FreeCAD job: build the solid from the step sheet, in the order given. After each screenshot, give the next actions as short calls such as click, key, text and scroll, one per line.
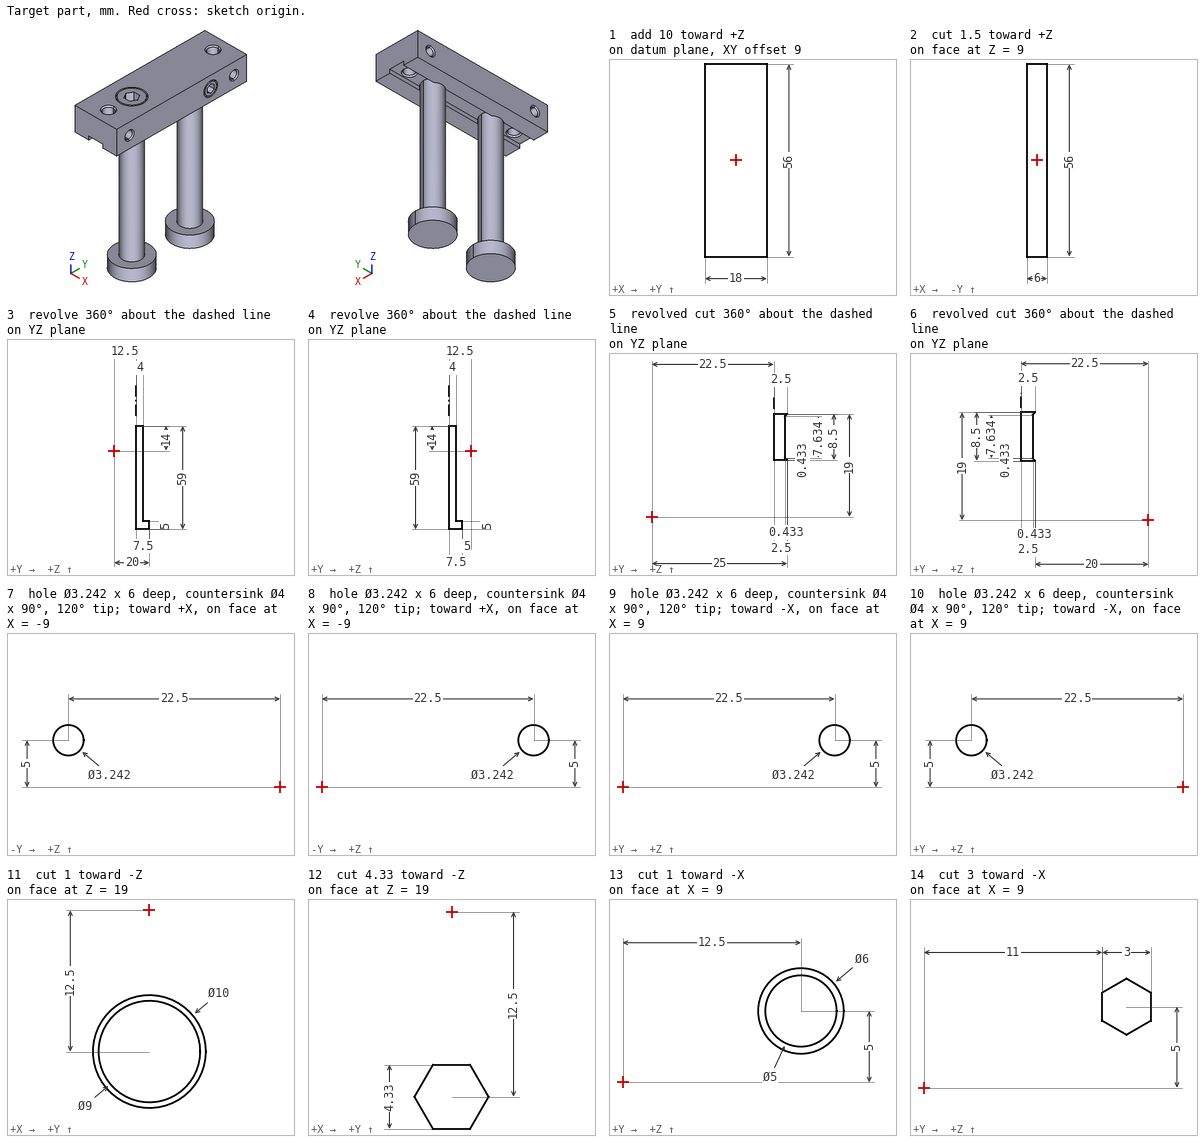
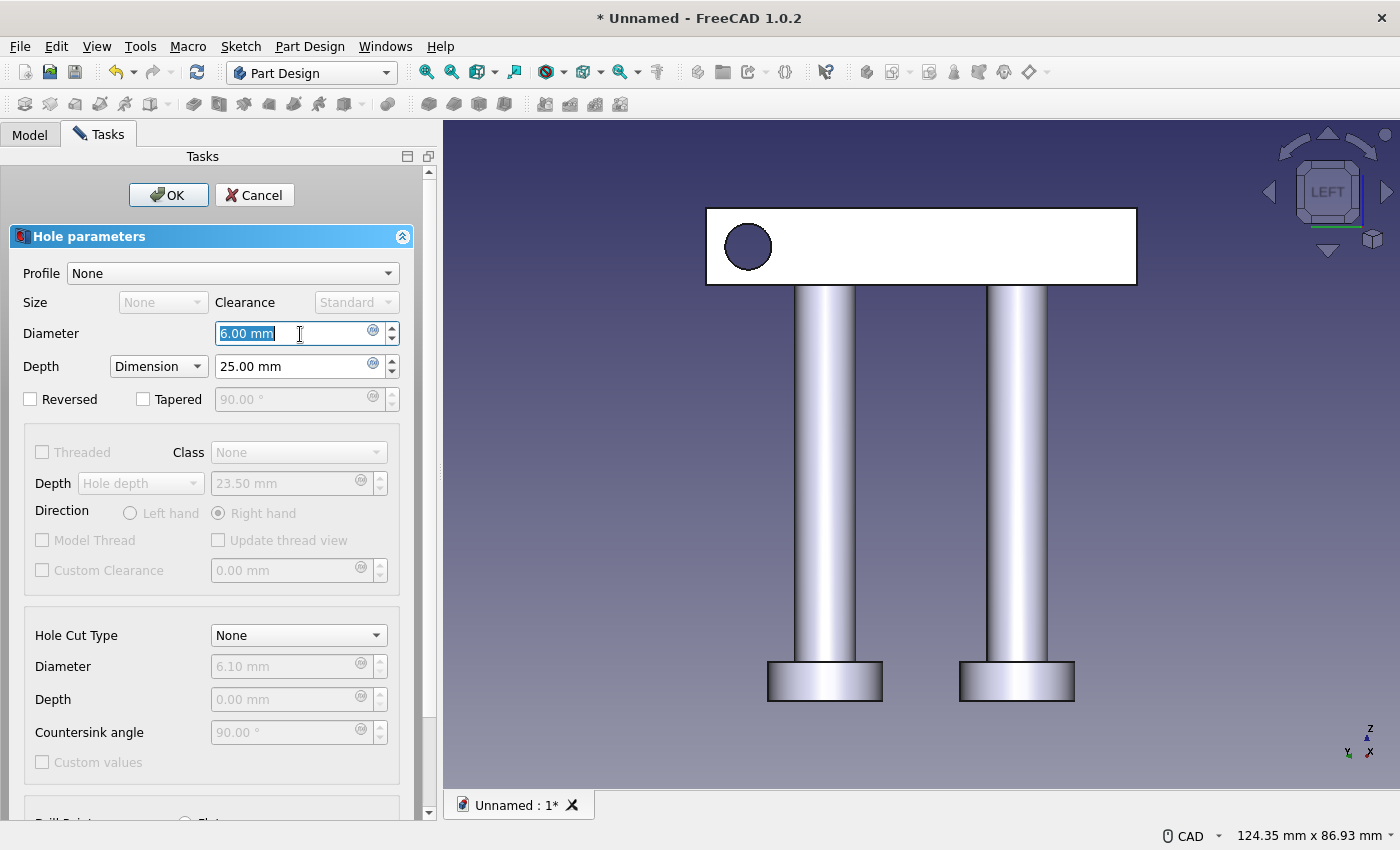
text(3.242)
key(Tab)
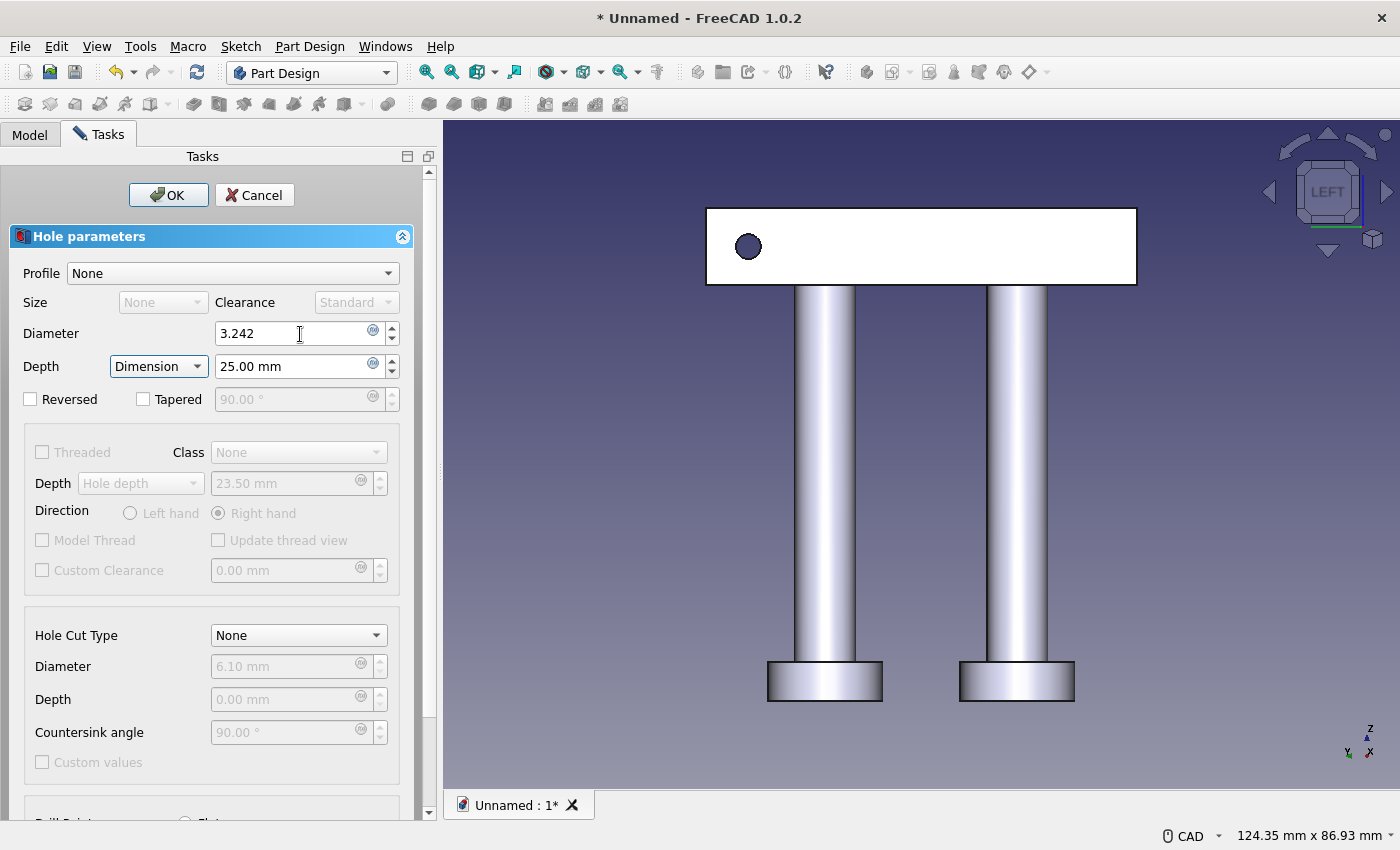
triple_click(300, 366)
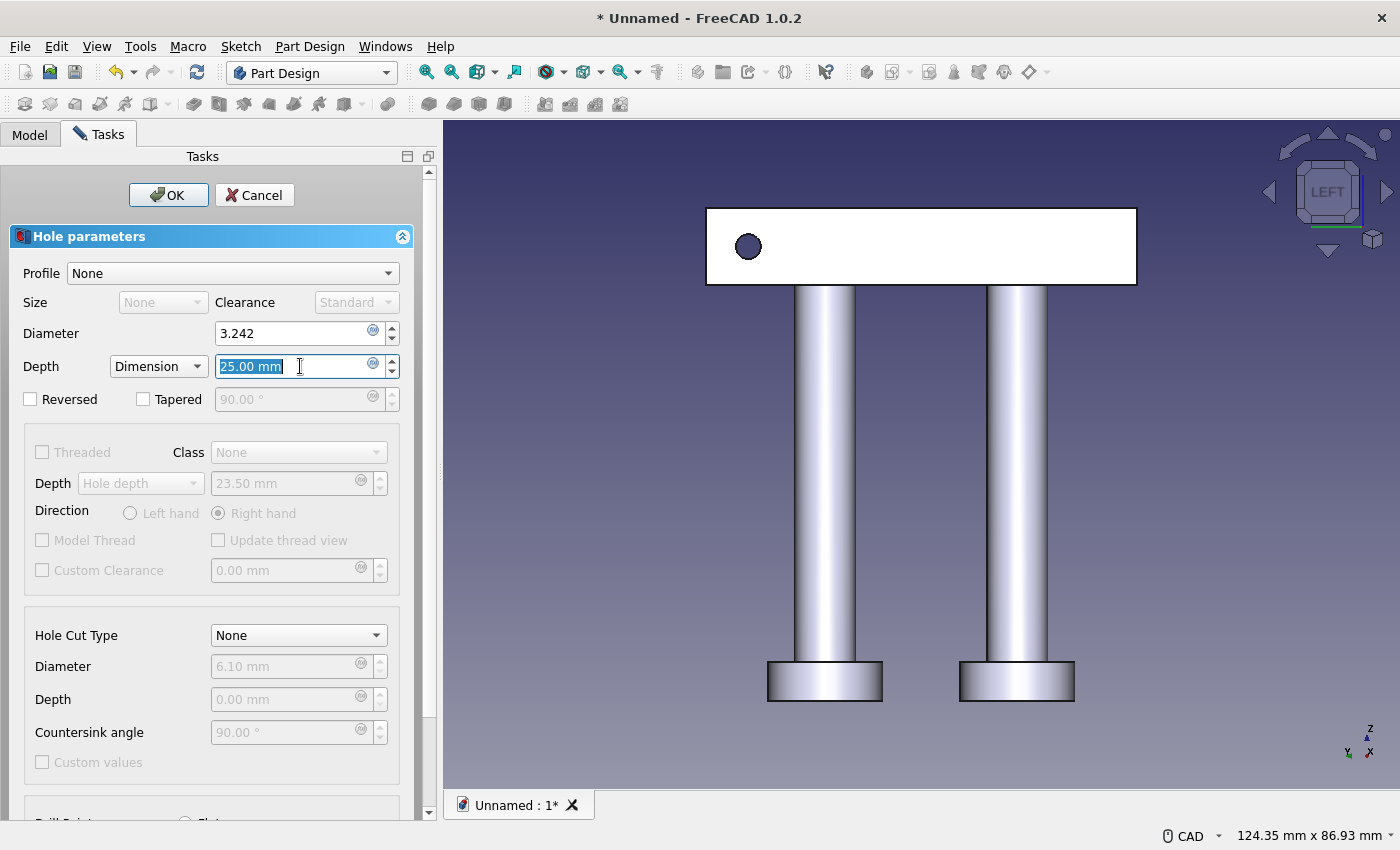
text(6)
key(Tab)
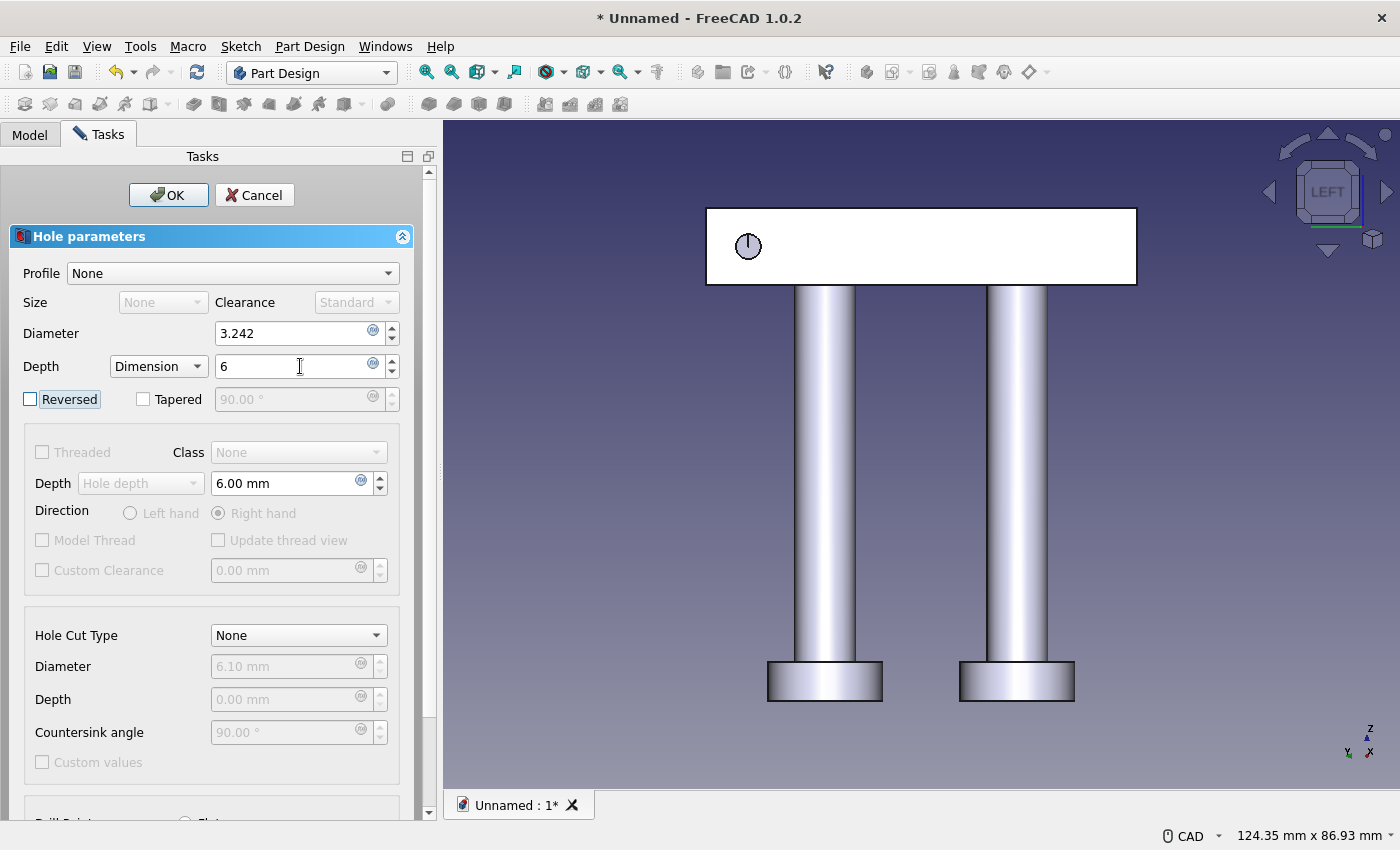
click(300, 636)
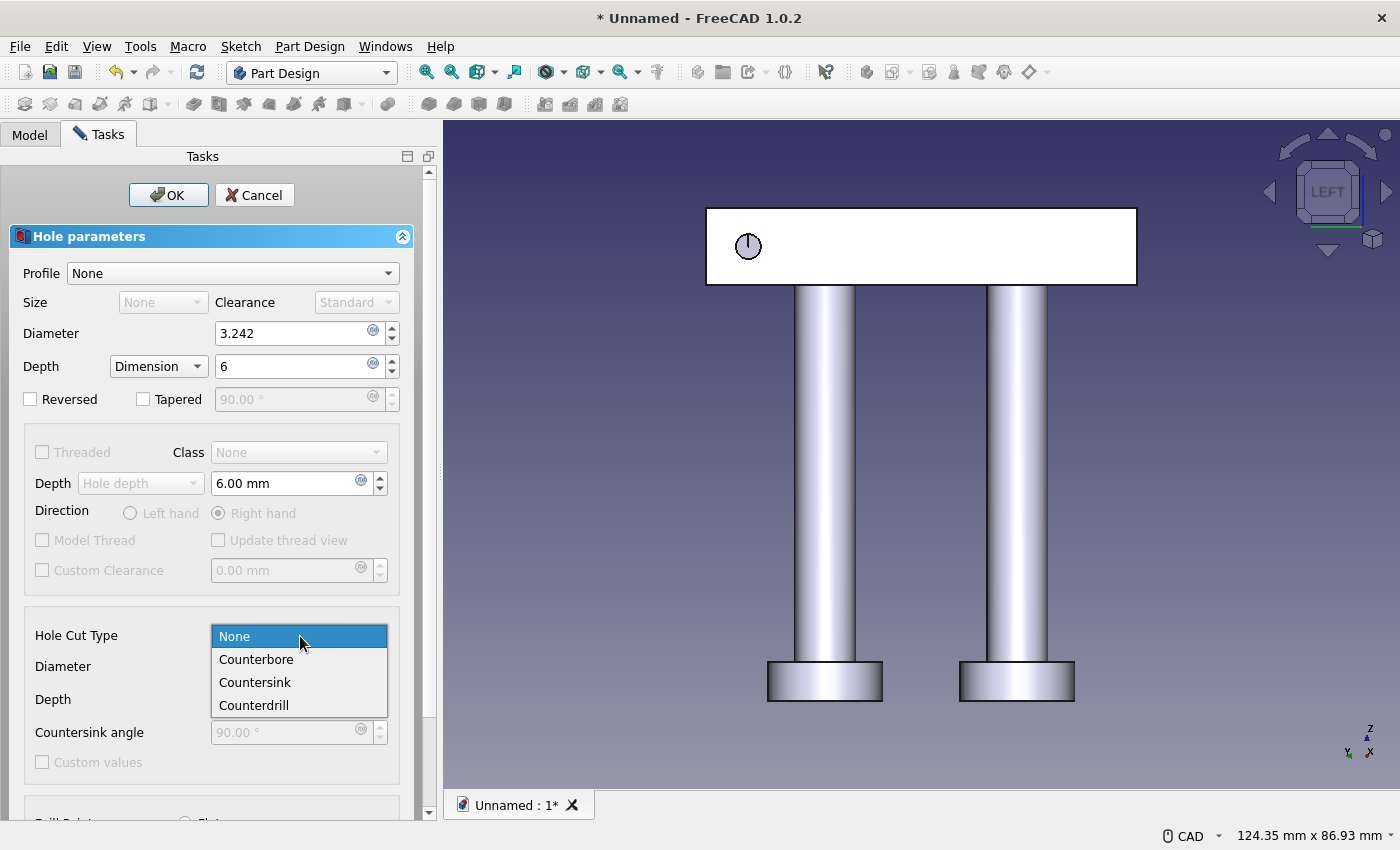
click(298, 682)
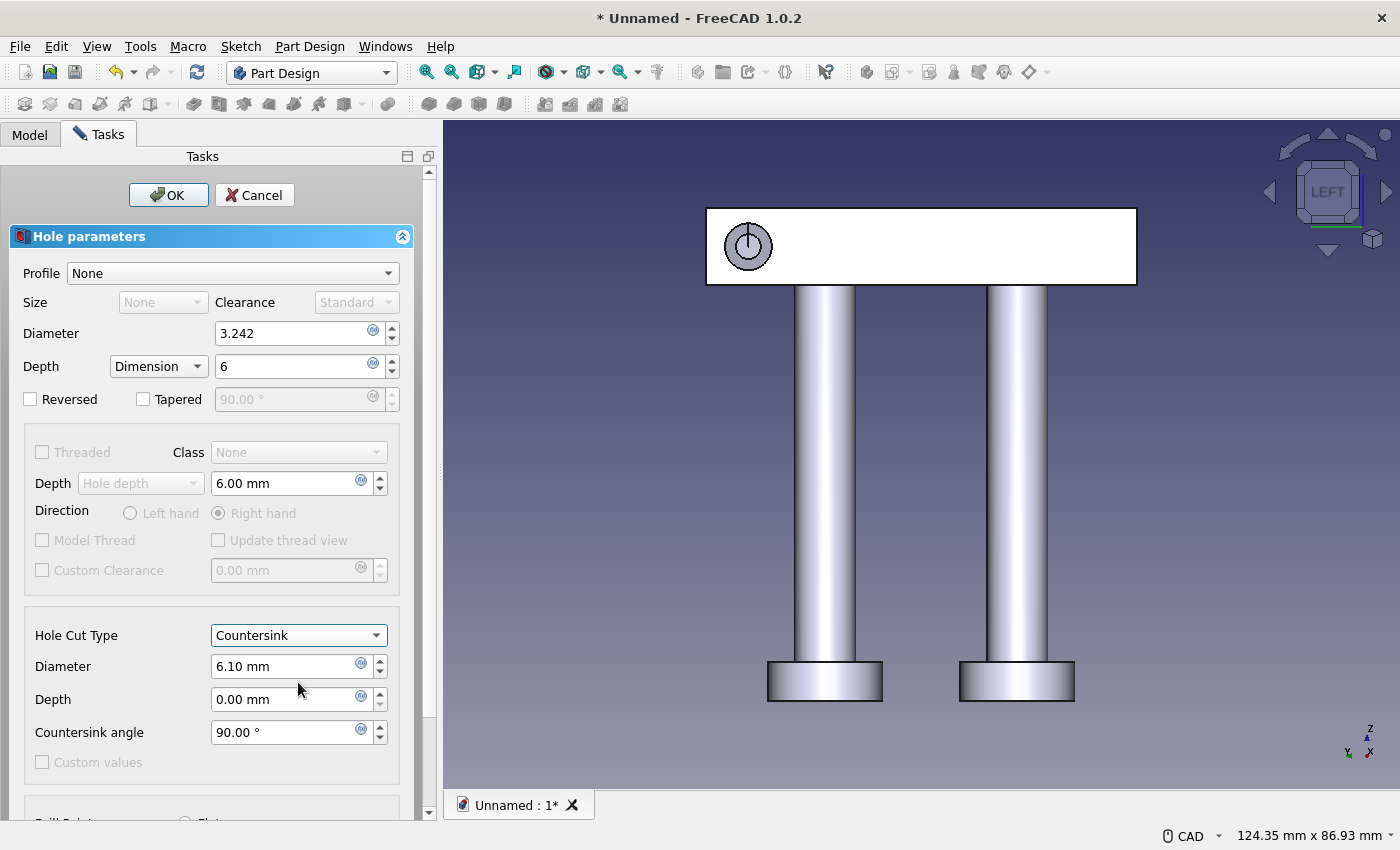
triple_click(292, 666)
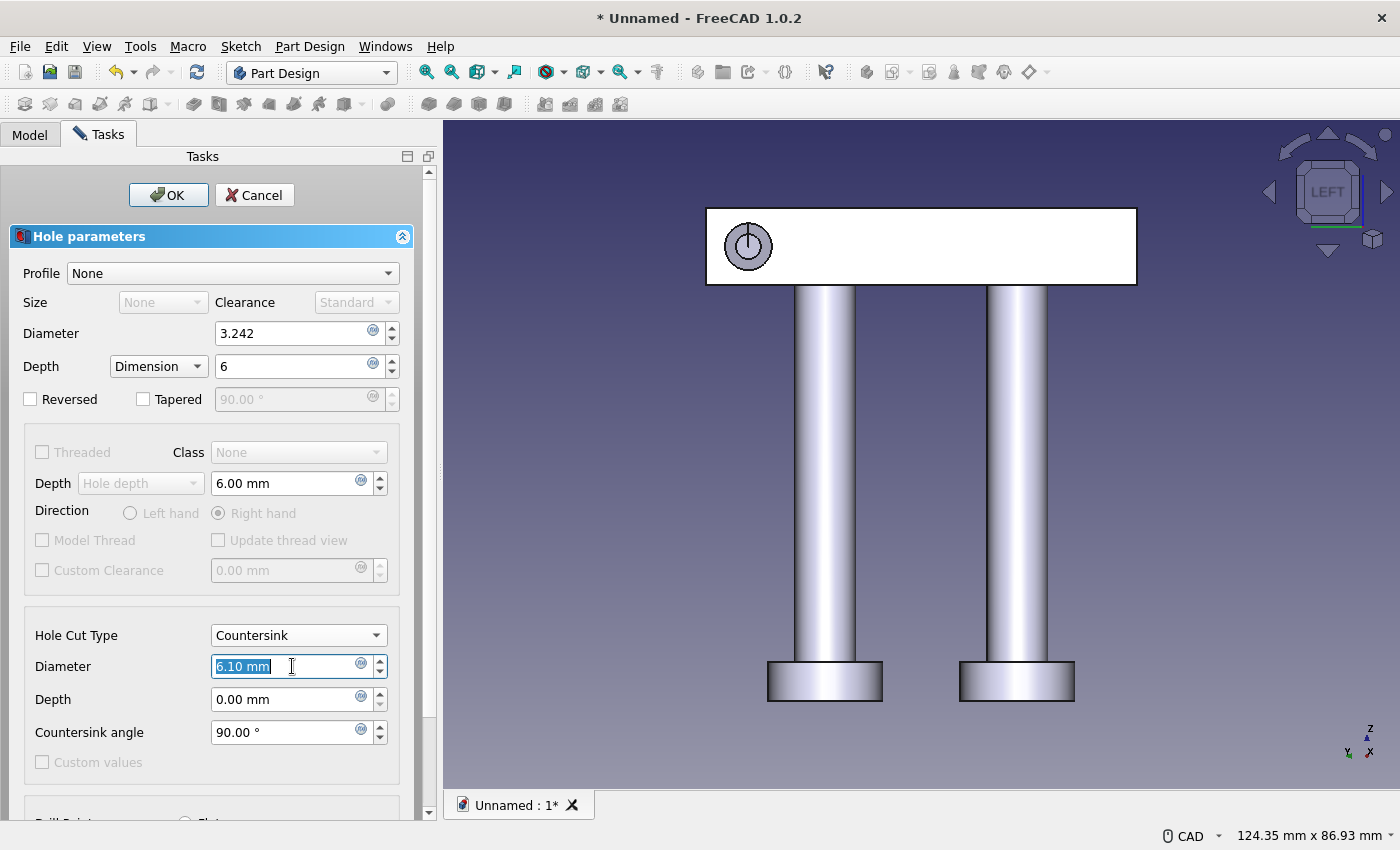
text(4)
key(Tab)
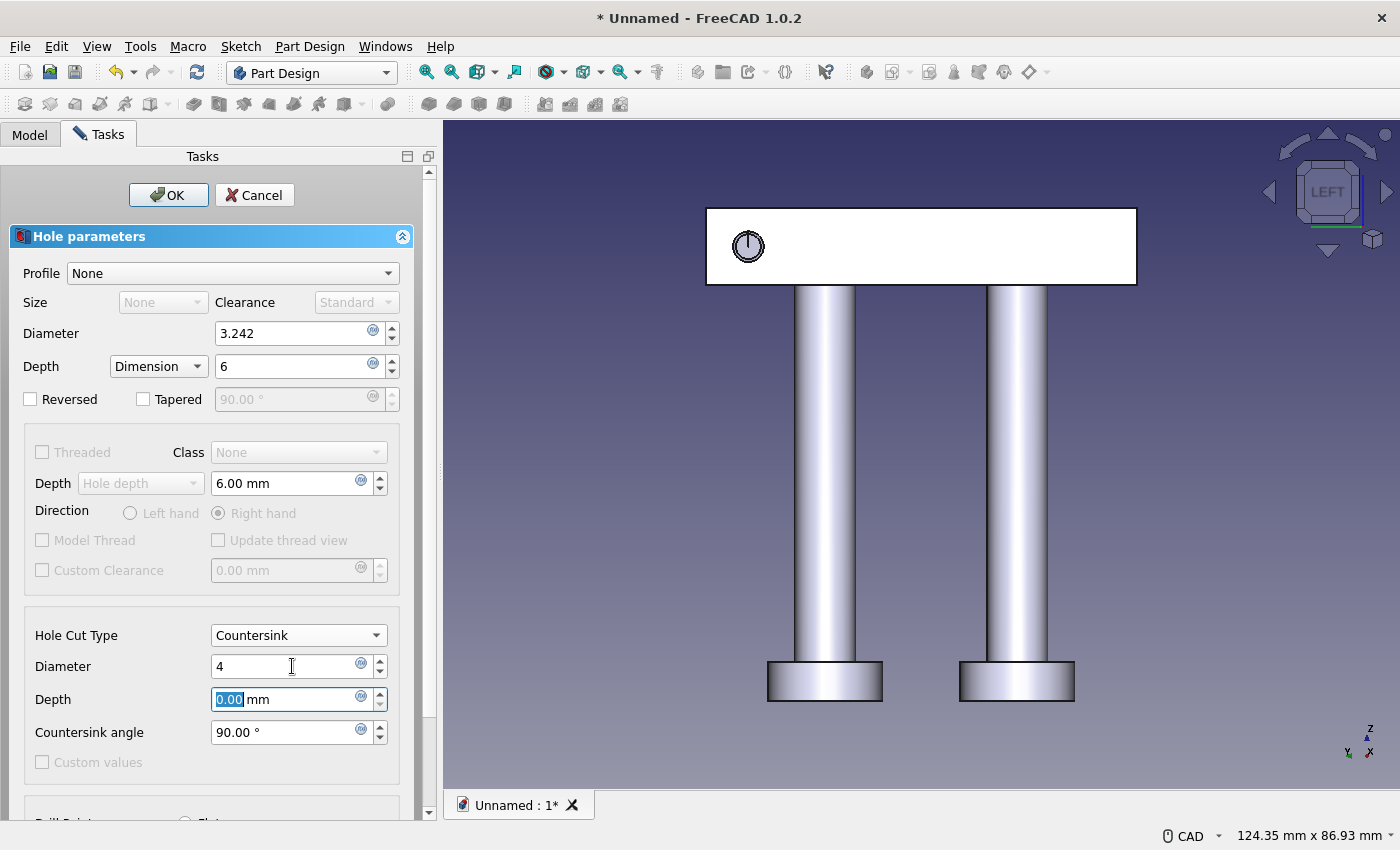
scroll(429, 493, down, 2)